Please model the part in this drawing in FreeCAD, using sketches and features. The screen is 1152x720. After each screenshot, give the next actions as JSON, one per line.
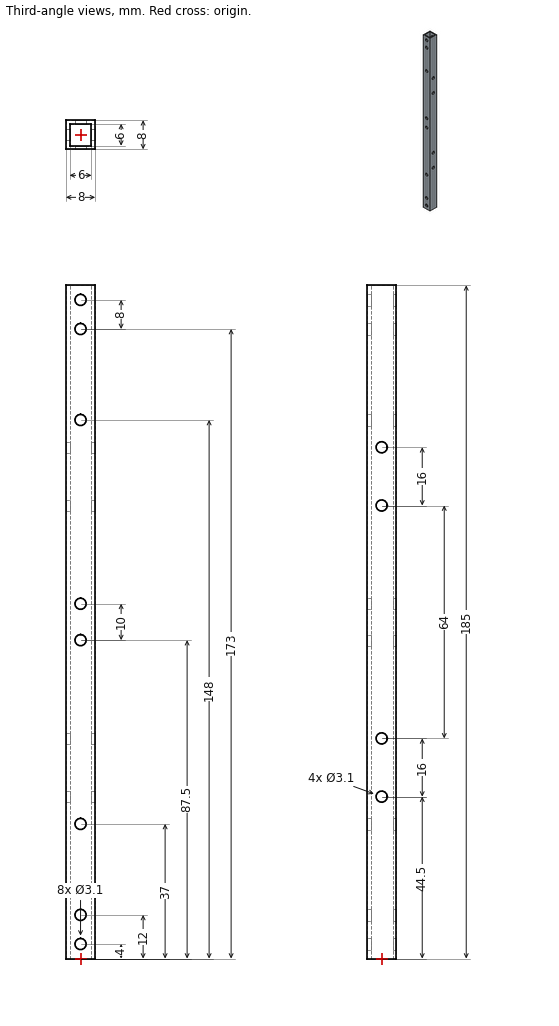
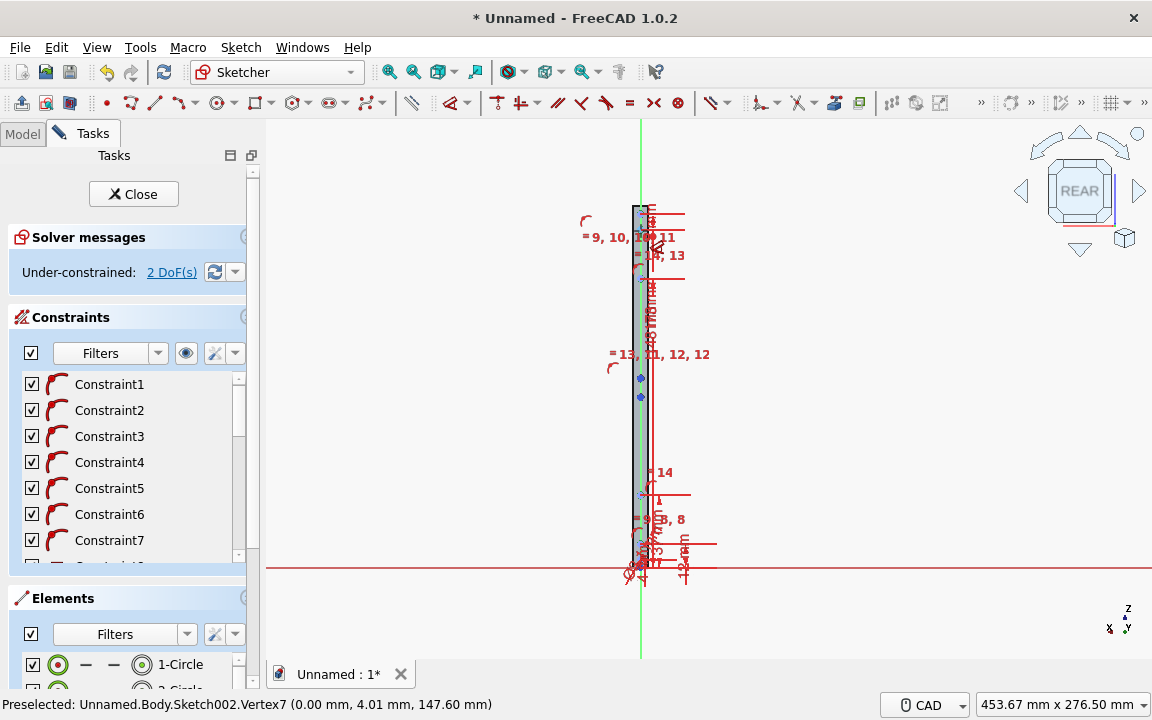
{"action": "scroll", "coordinate": [641, 397], "scroll_direction": "up", "scroll_amount": 4}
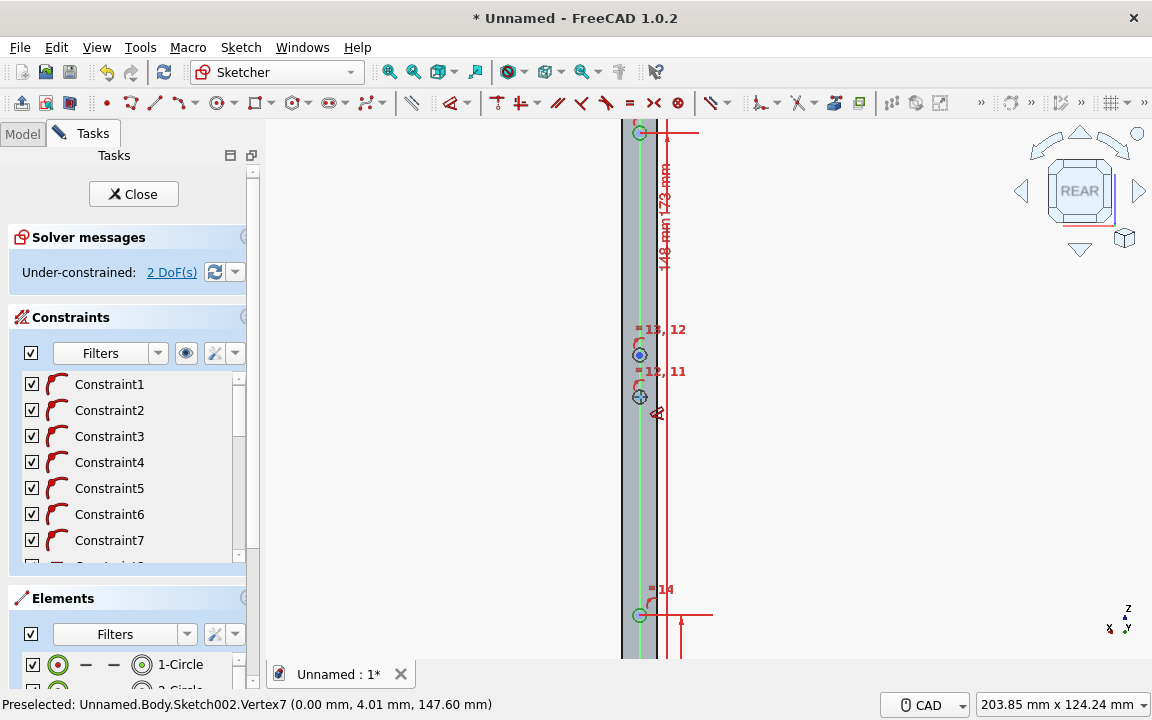
{"action": "left_click", "coordinate": [640, 397]}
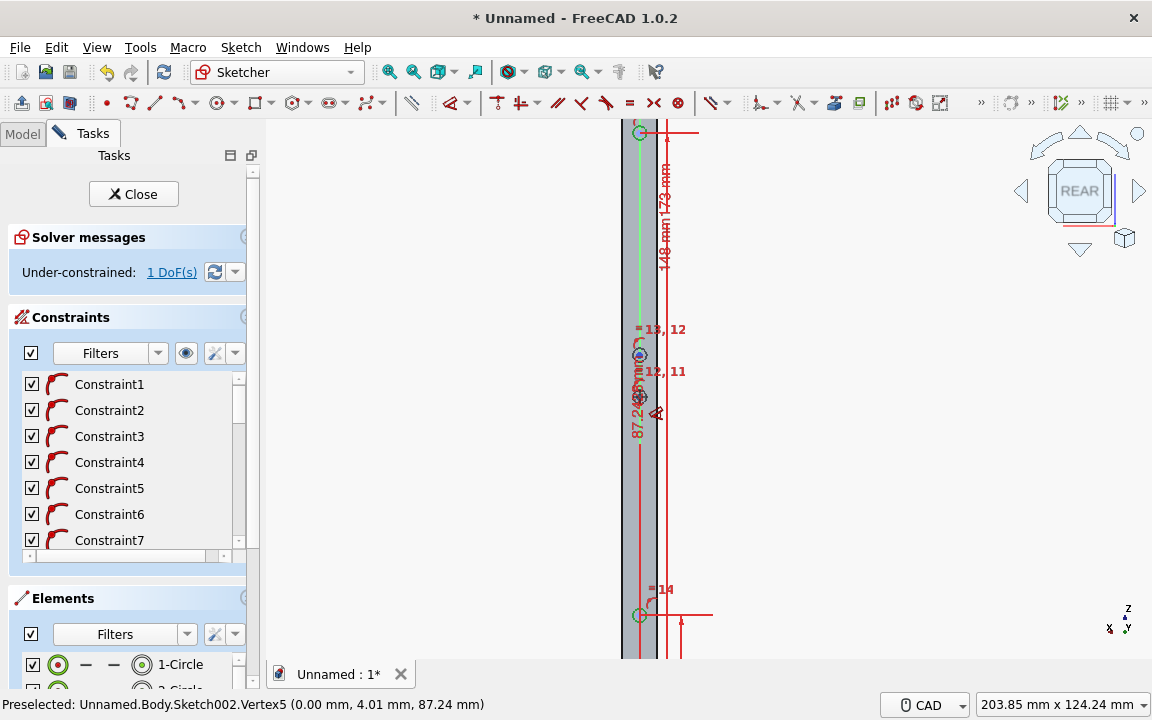
{"action": "left_click", "coordinate": [640, 355]}
{"action": "left_click", "coordinate": [674, 376]}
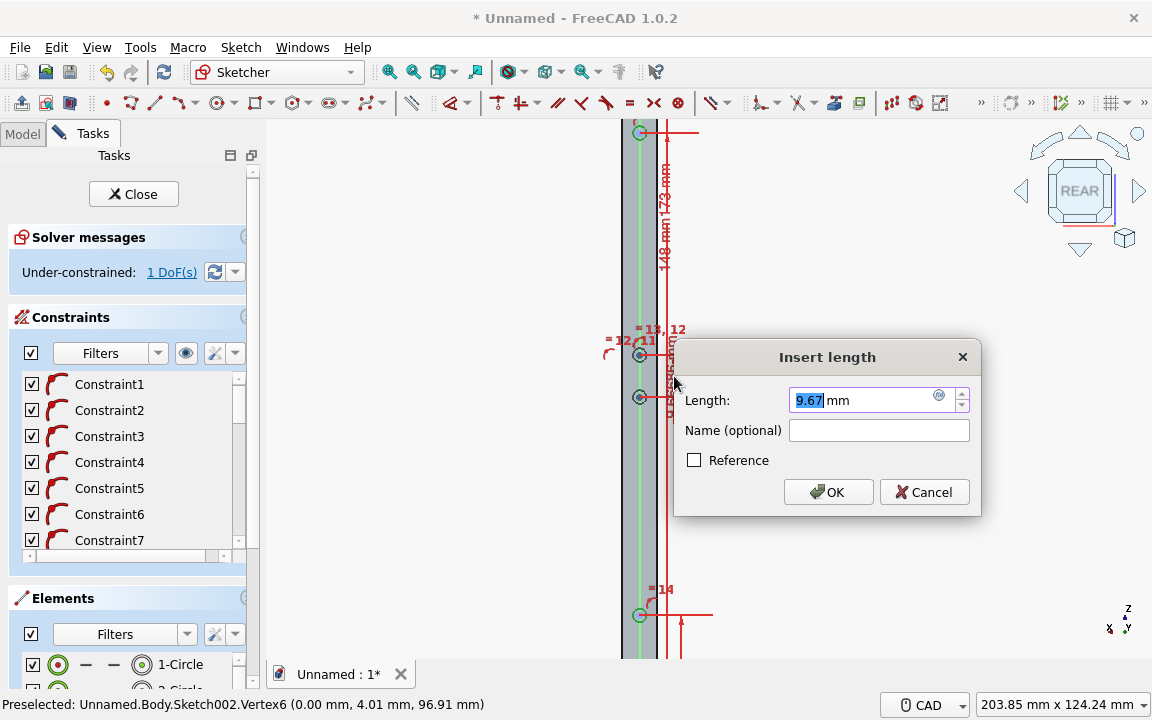
{"action": "type", "text": "10"}
{"action": "key", "text": "Return"}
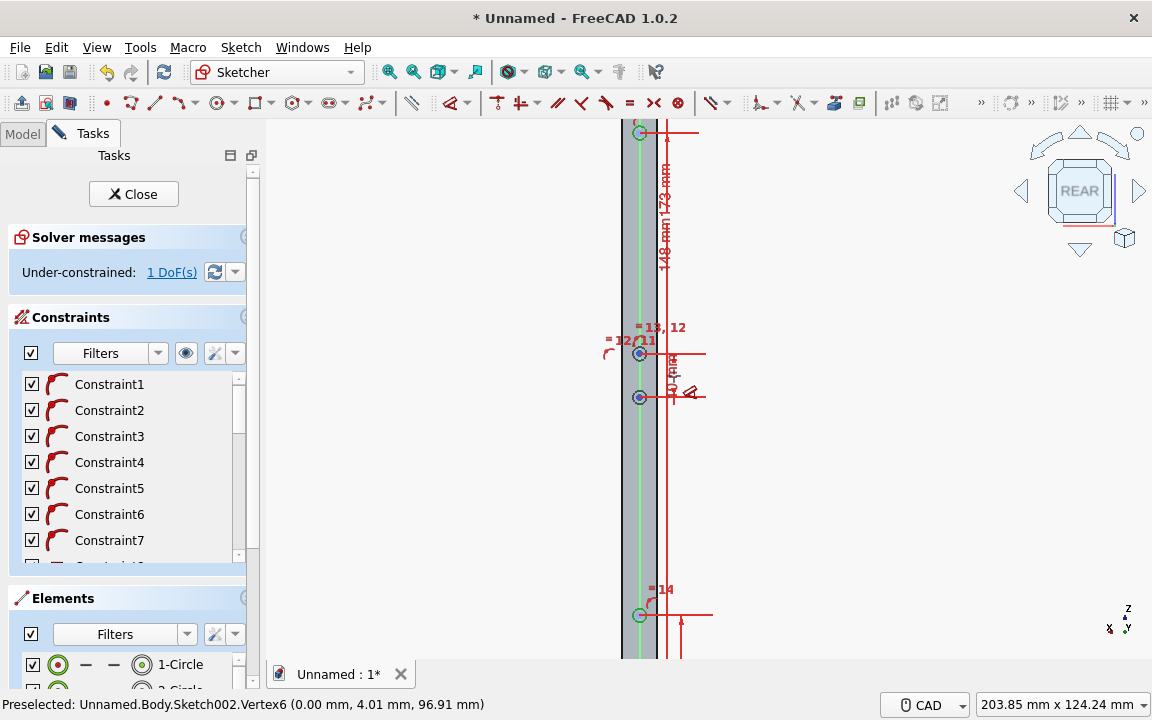
{"action": "left_click", "coordinate": [640, 397]}
{"action": "left_click", "coordinate": [674, 514]}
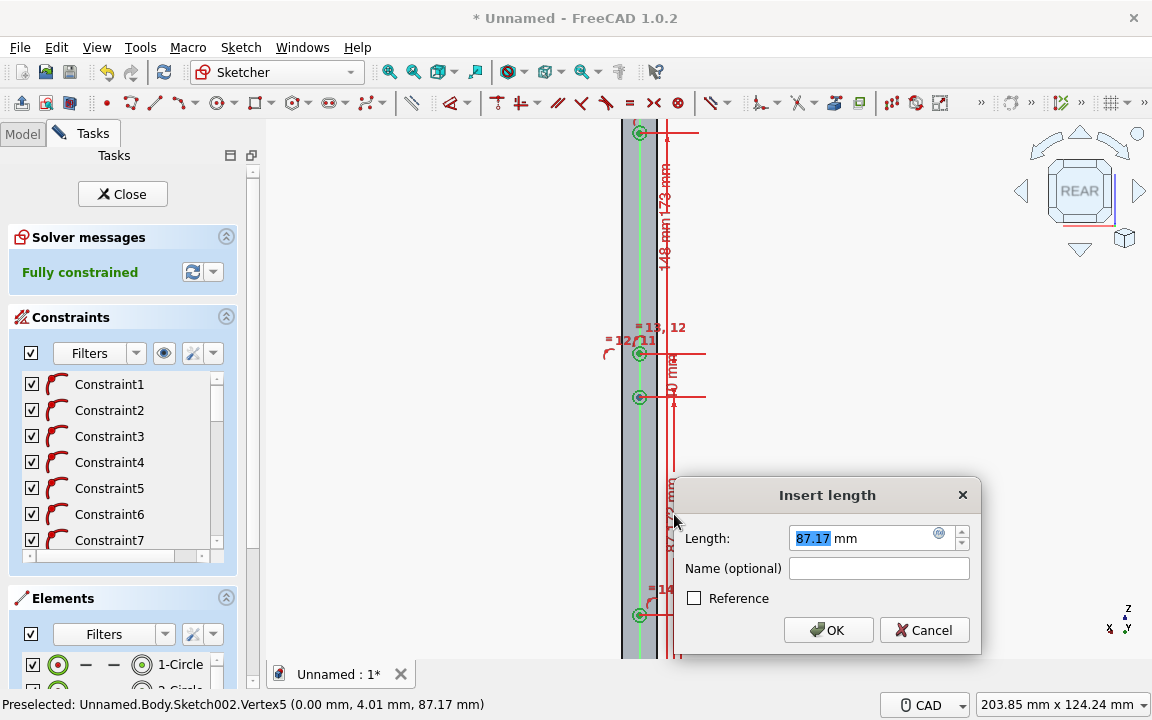
{"action": "type", "text": "87.5"}
{"action": "key", "text": "Return"}
{"action": "key", "text": "Escape"}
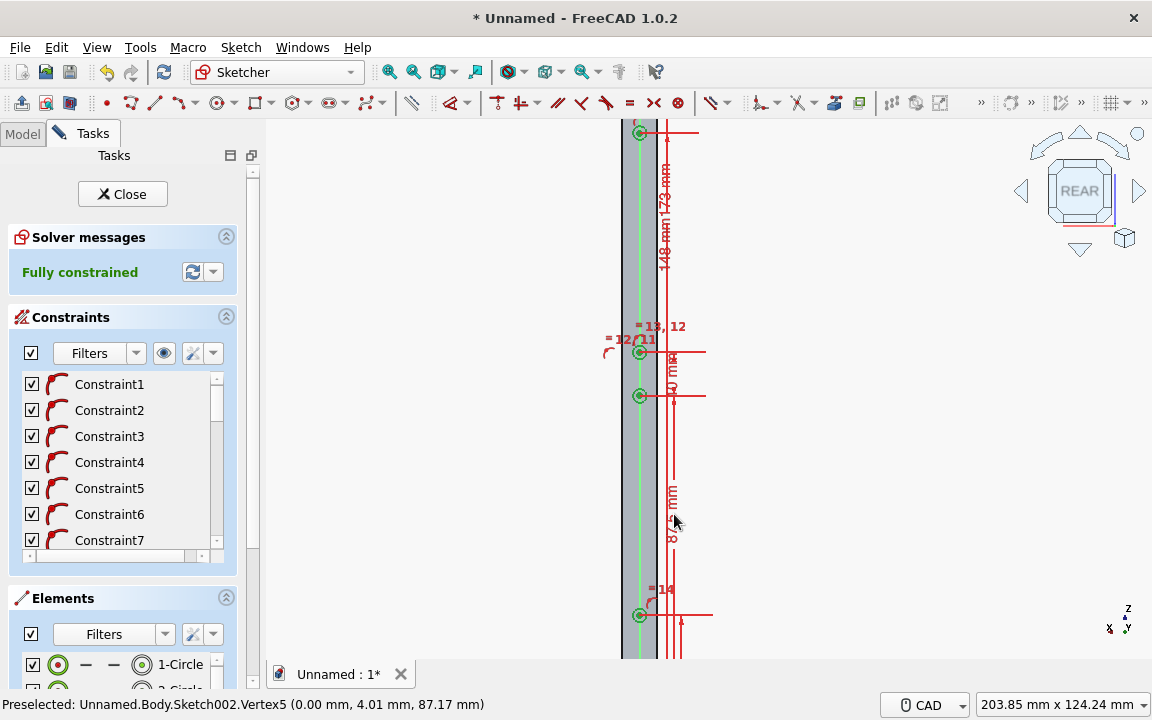
{"action": "left_click", "coordinate": [123, 194]}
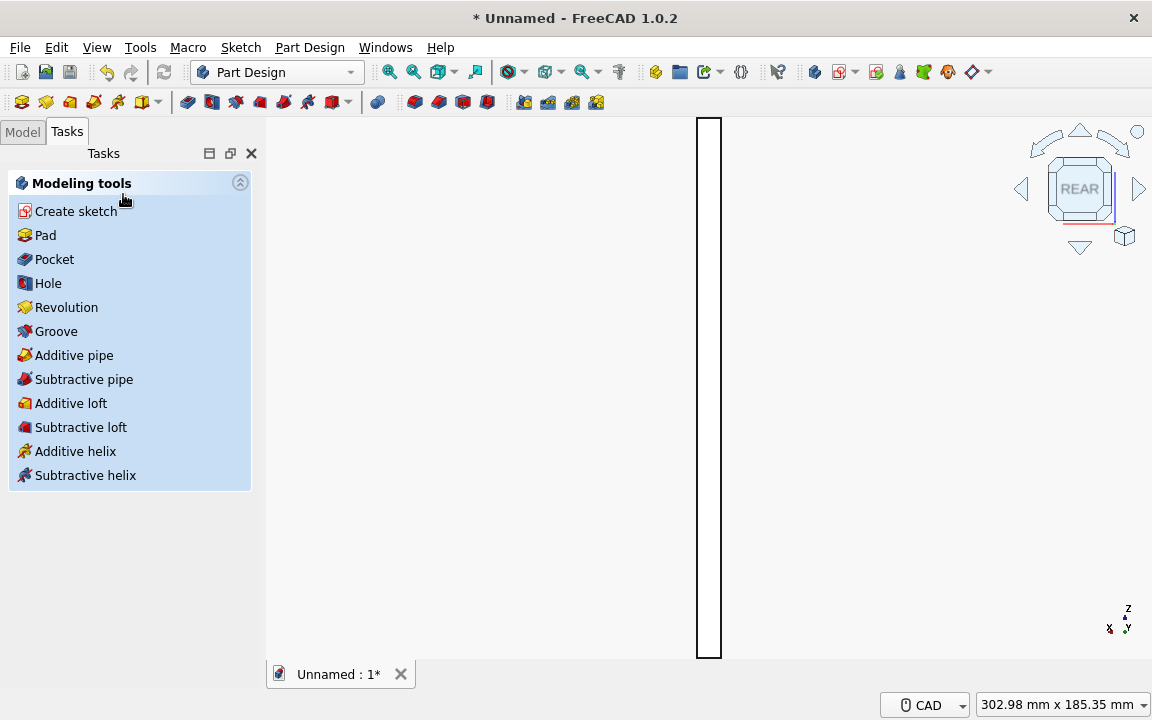
{"action": "left_click", "coordinate": [188, 102]}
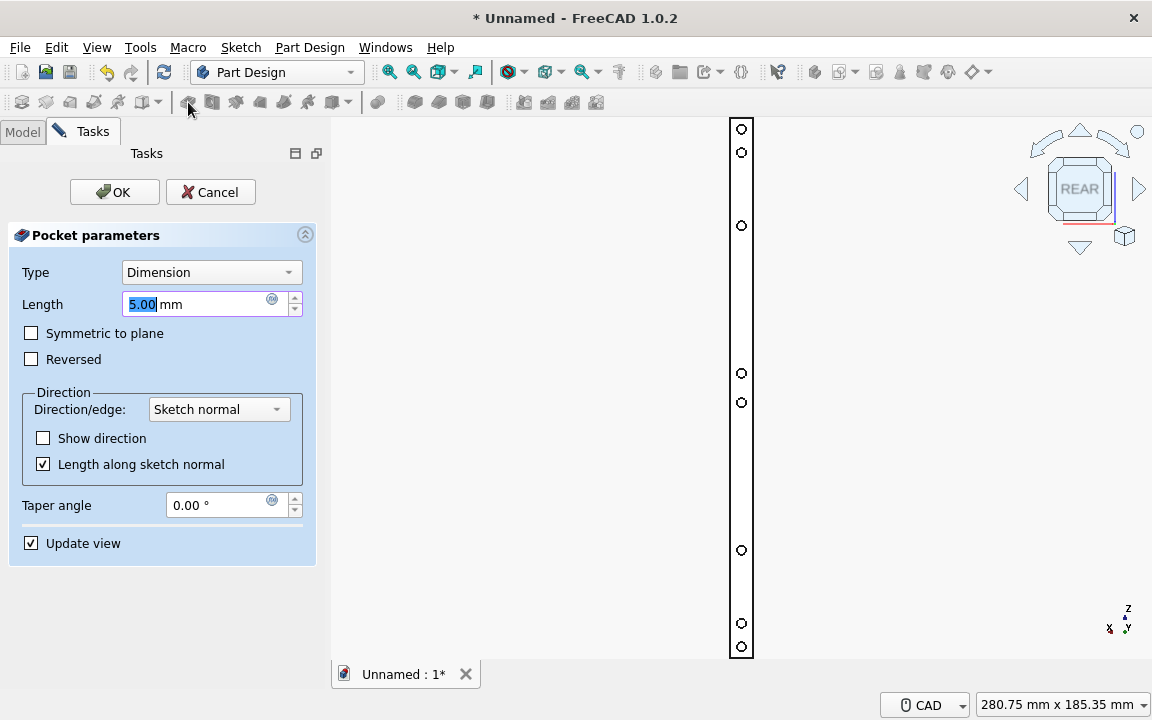
{"action": "left_click", "coordinate": [212, 272]}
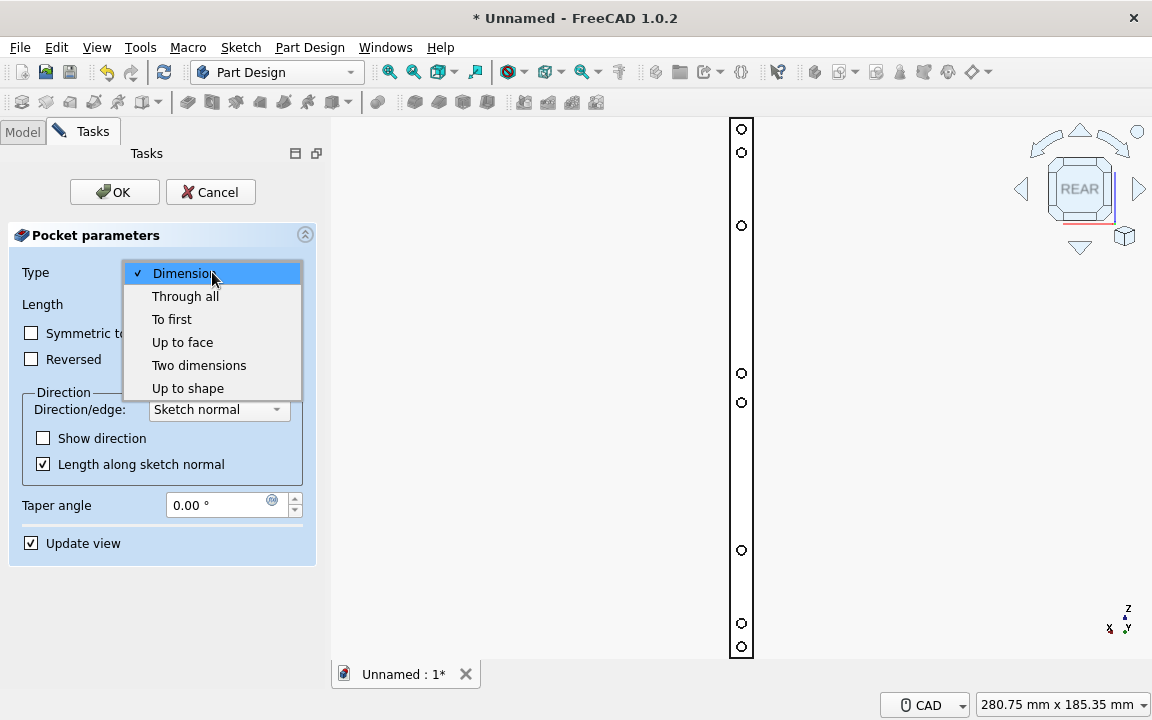
{"action": "left_click", "coordinate": [212, 296]}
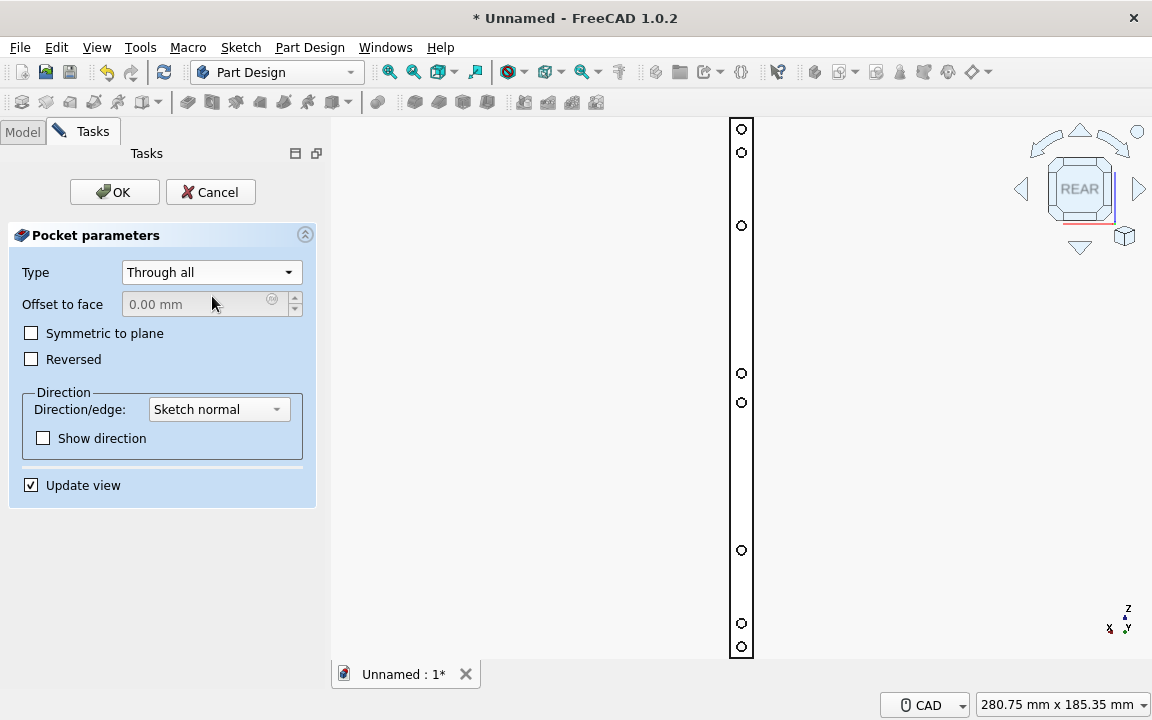
{"action": "left_click", "coordinate": [115, 192]}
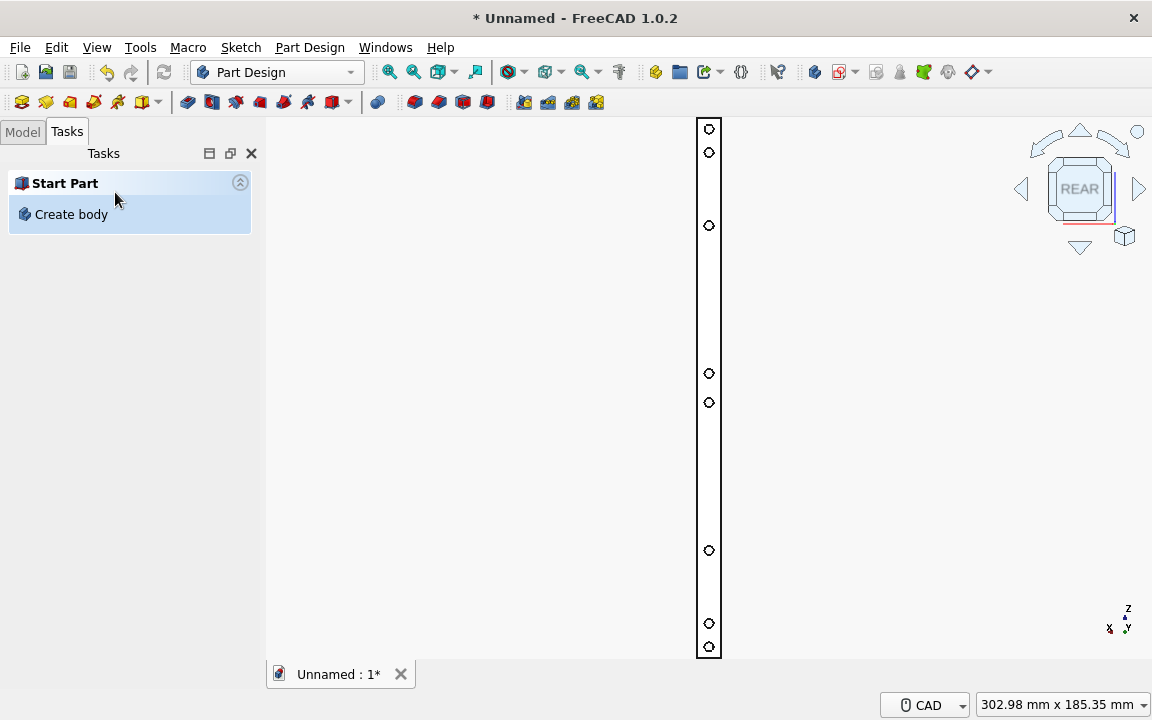
{"action": "key", "text": "0"}